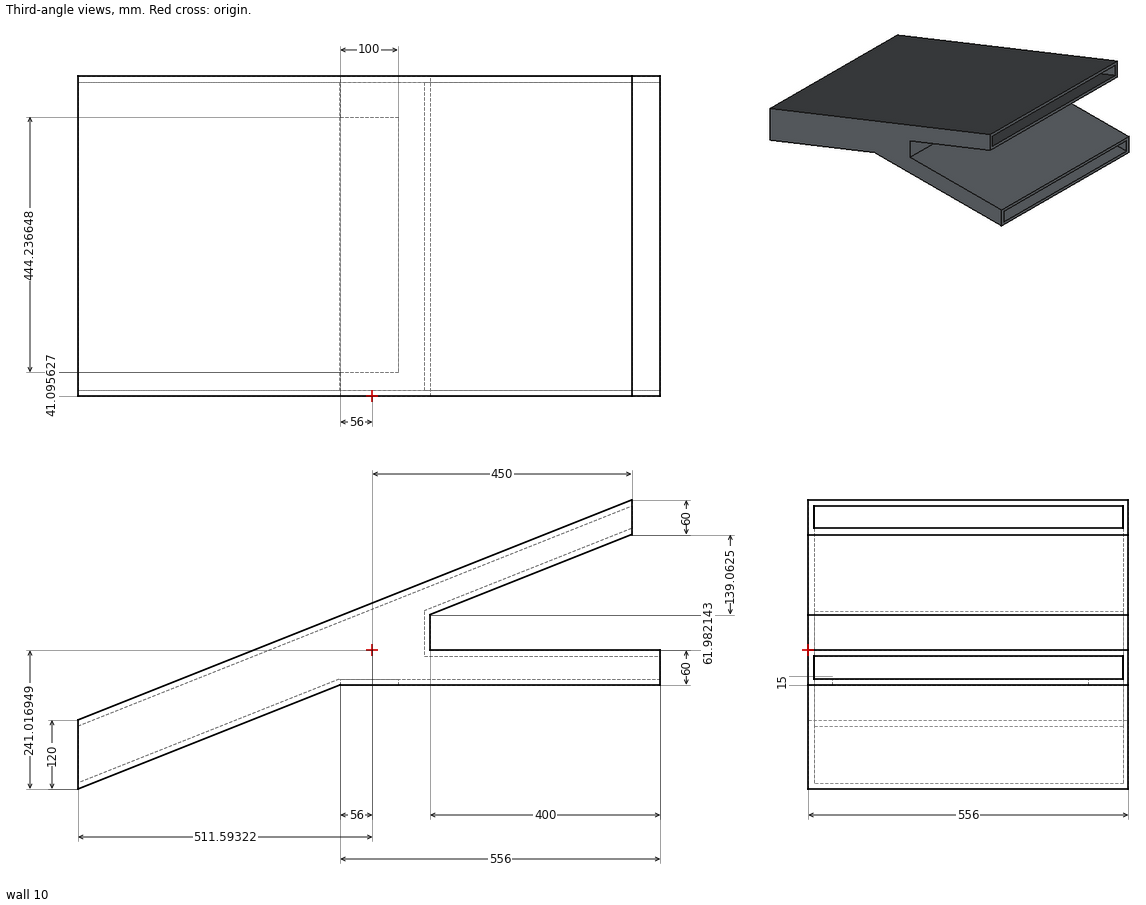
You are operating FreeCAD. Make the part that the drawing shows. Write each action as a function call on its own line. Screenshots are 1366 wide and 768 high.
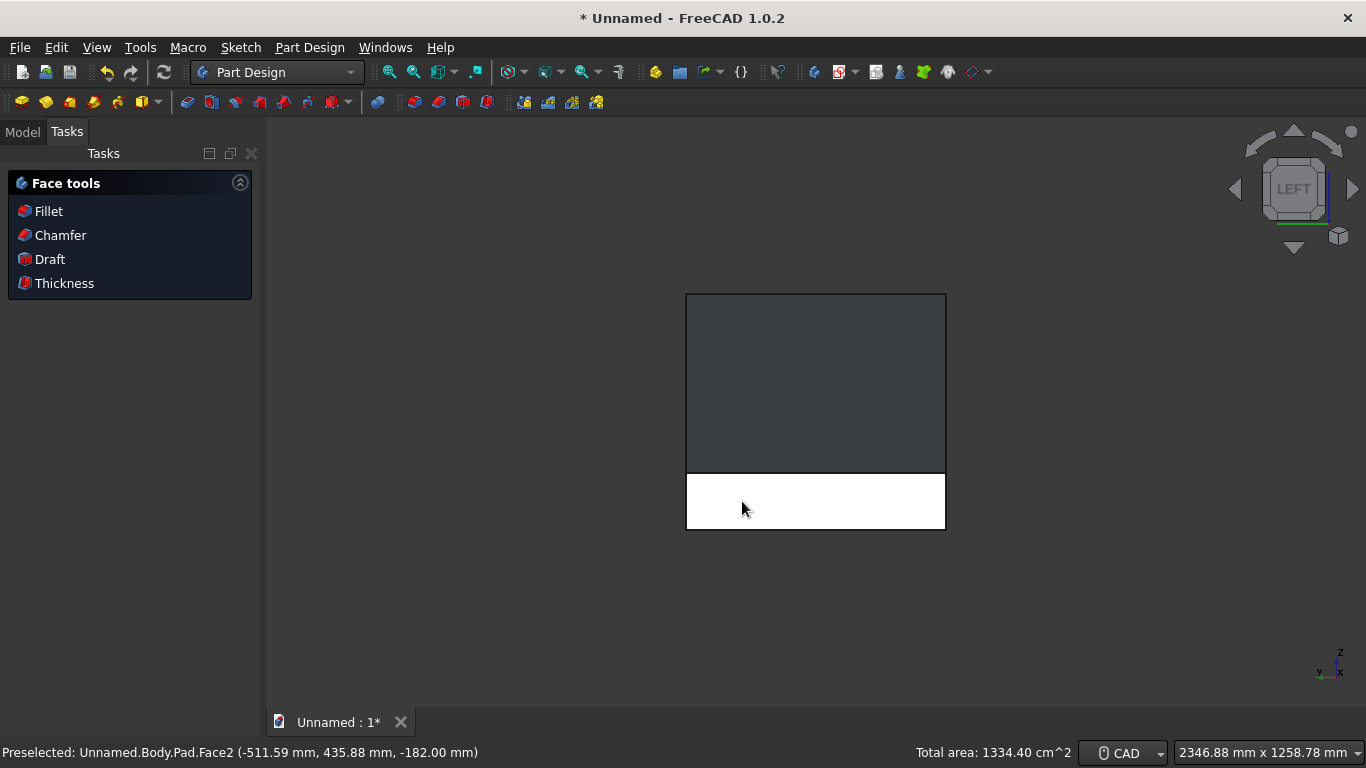
click(488, 102)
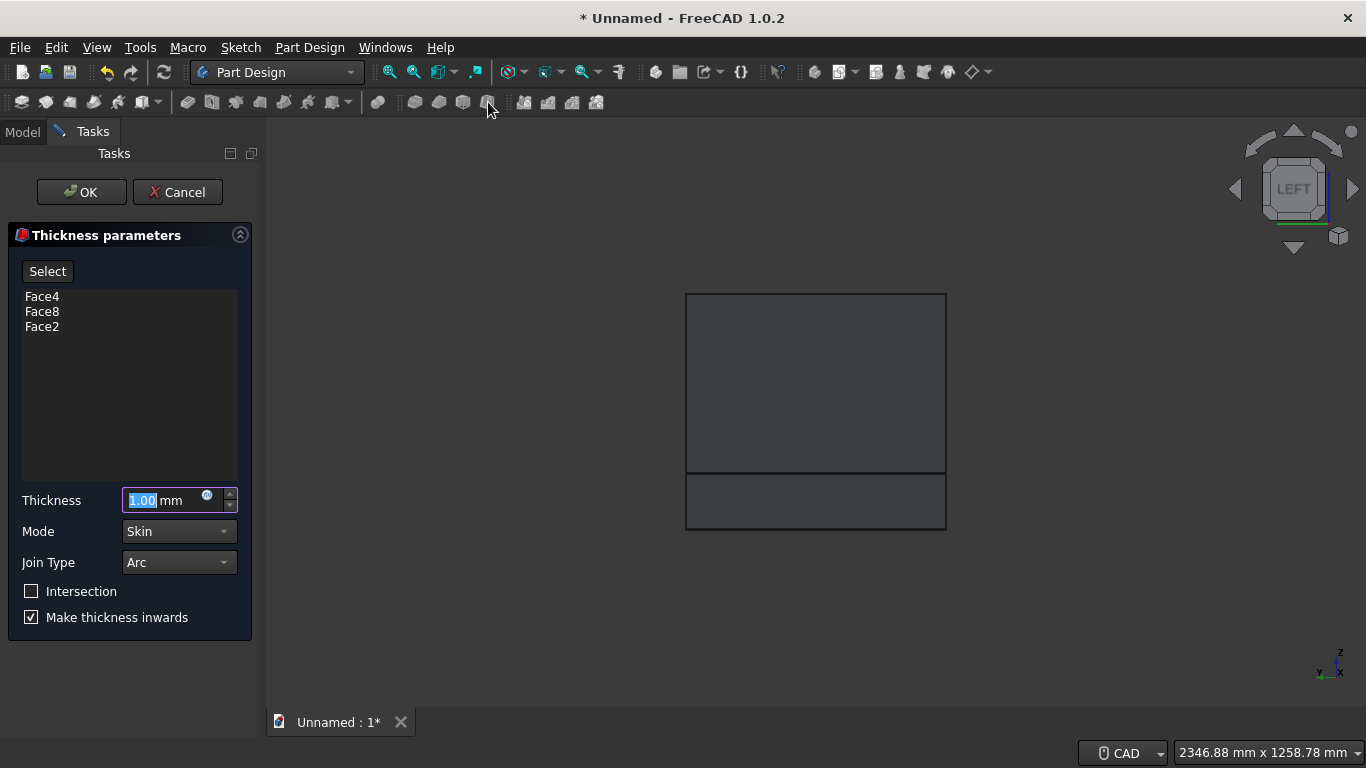
text(10)
key(Tab)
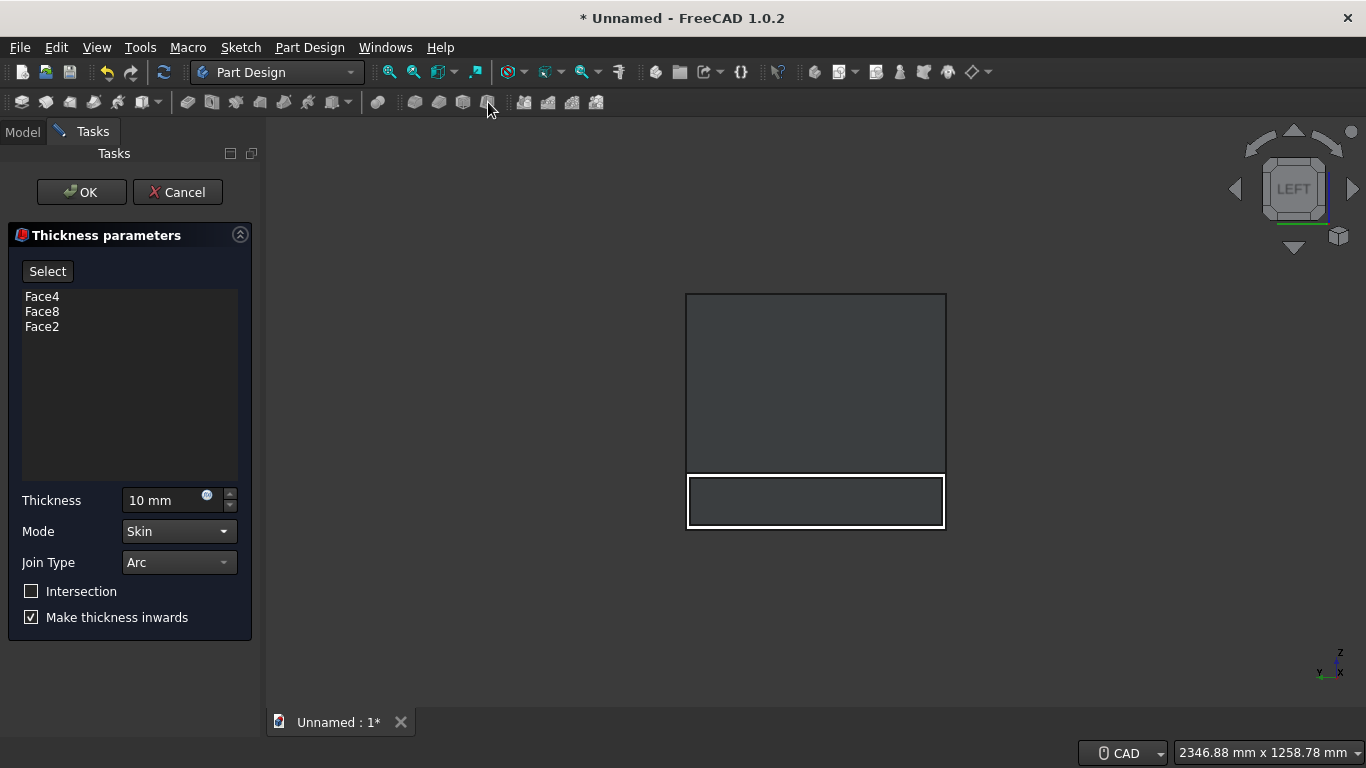
click(180, 562)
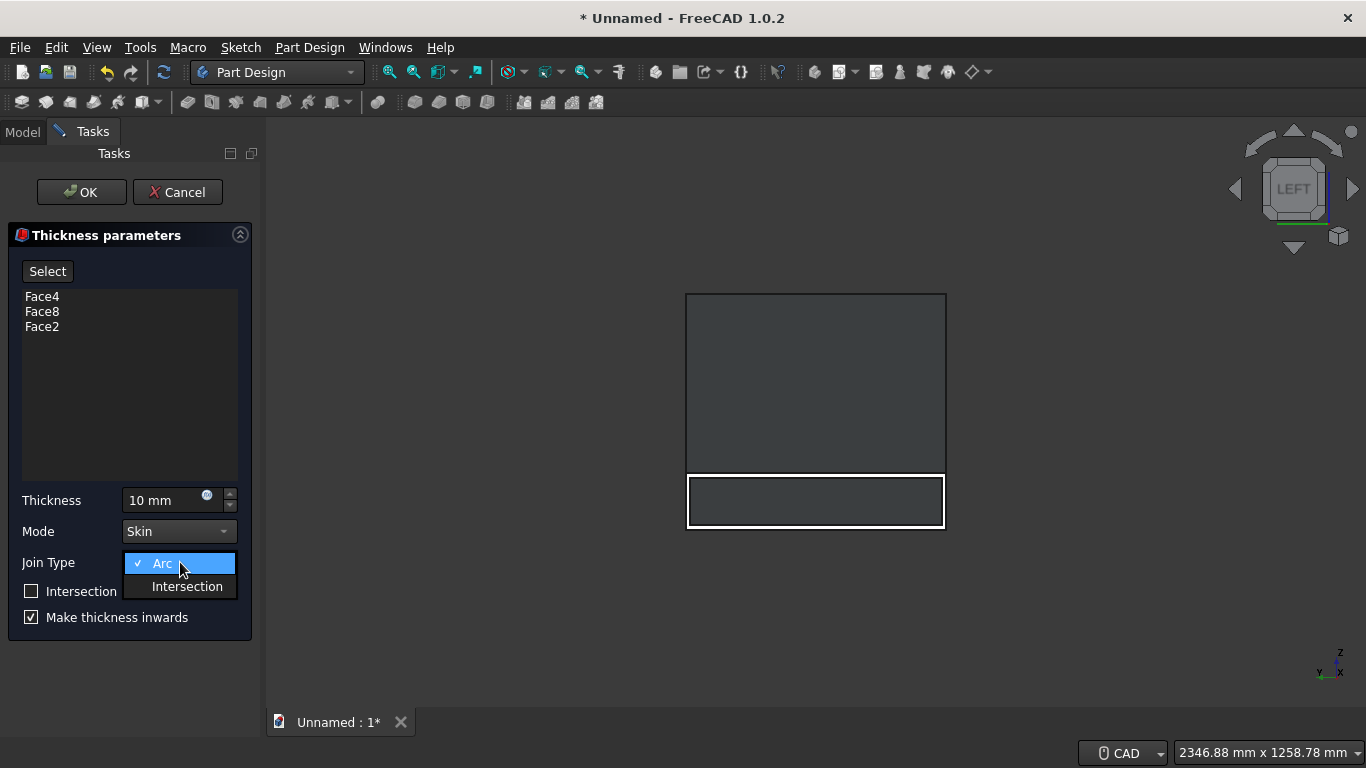
click(179, 586)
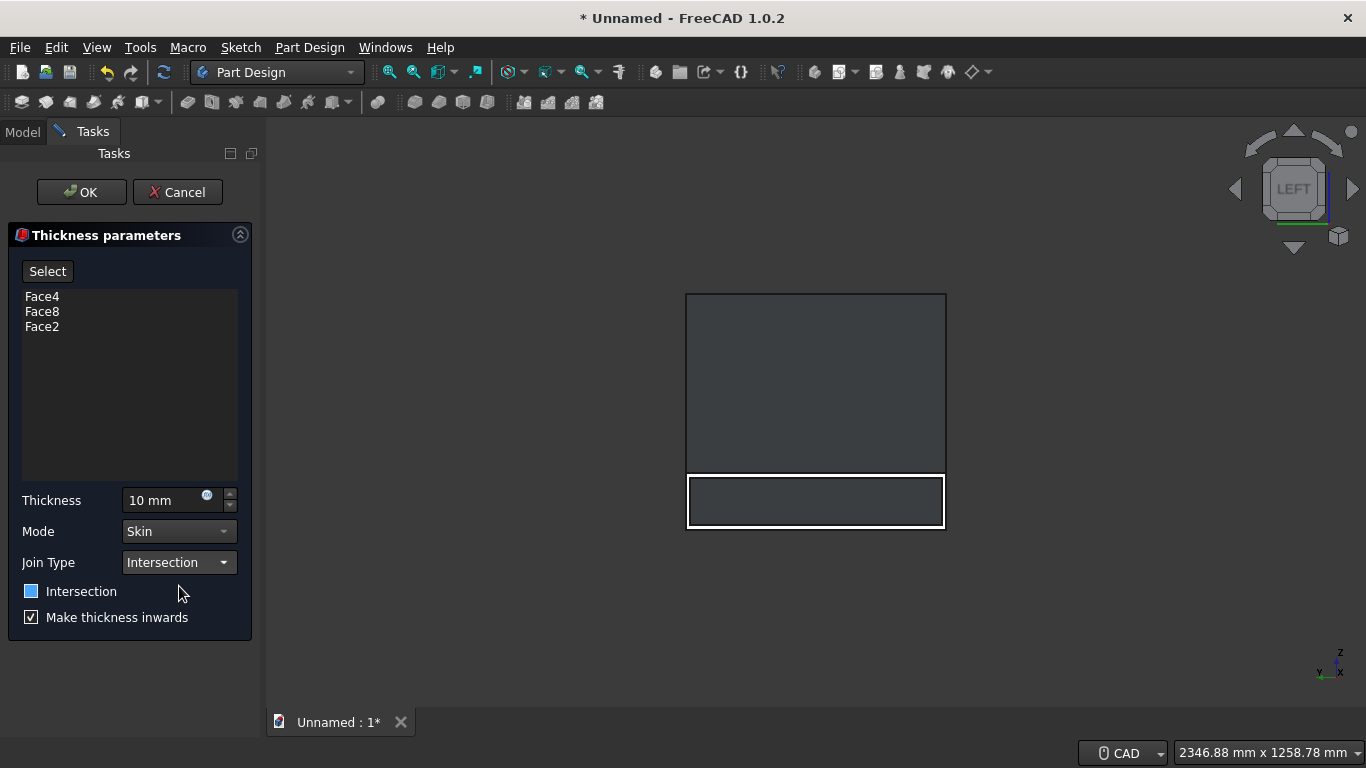
click(82, 192)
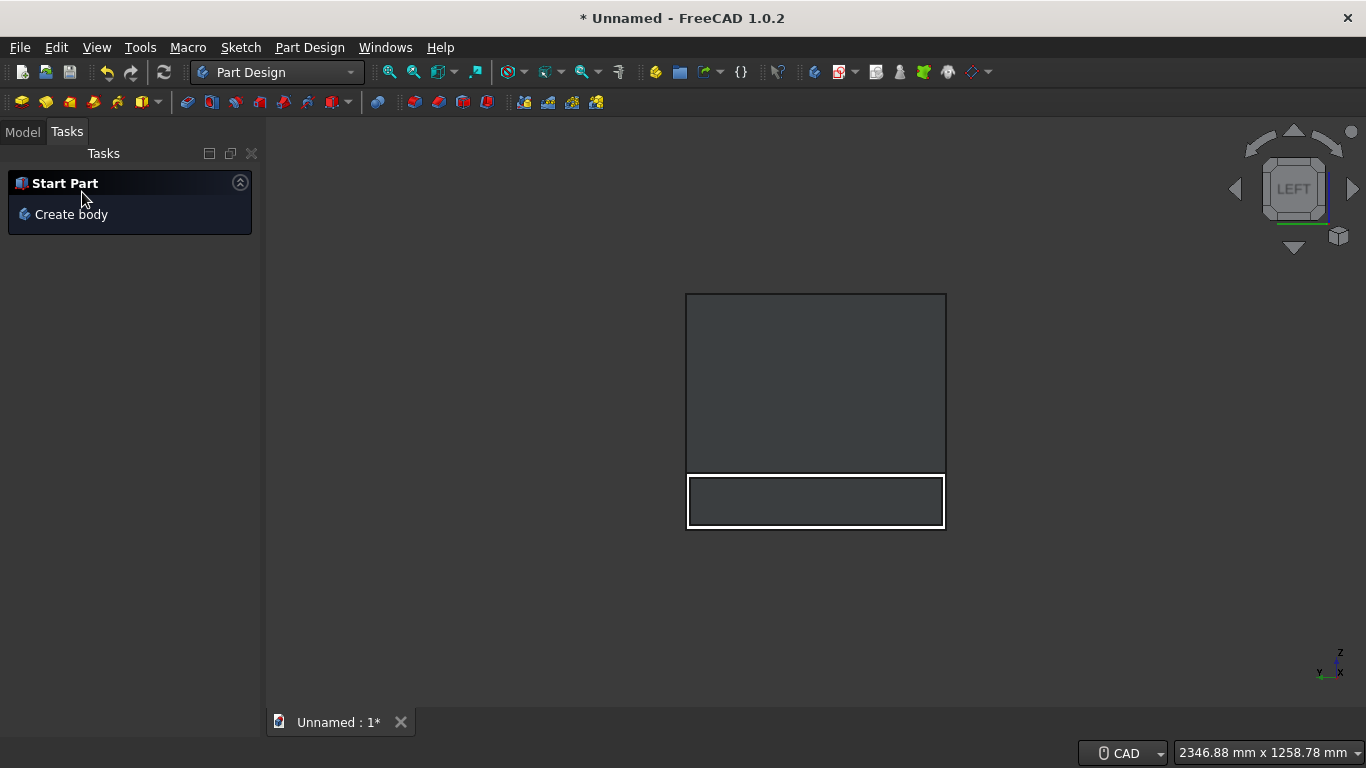
click(390, 72)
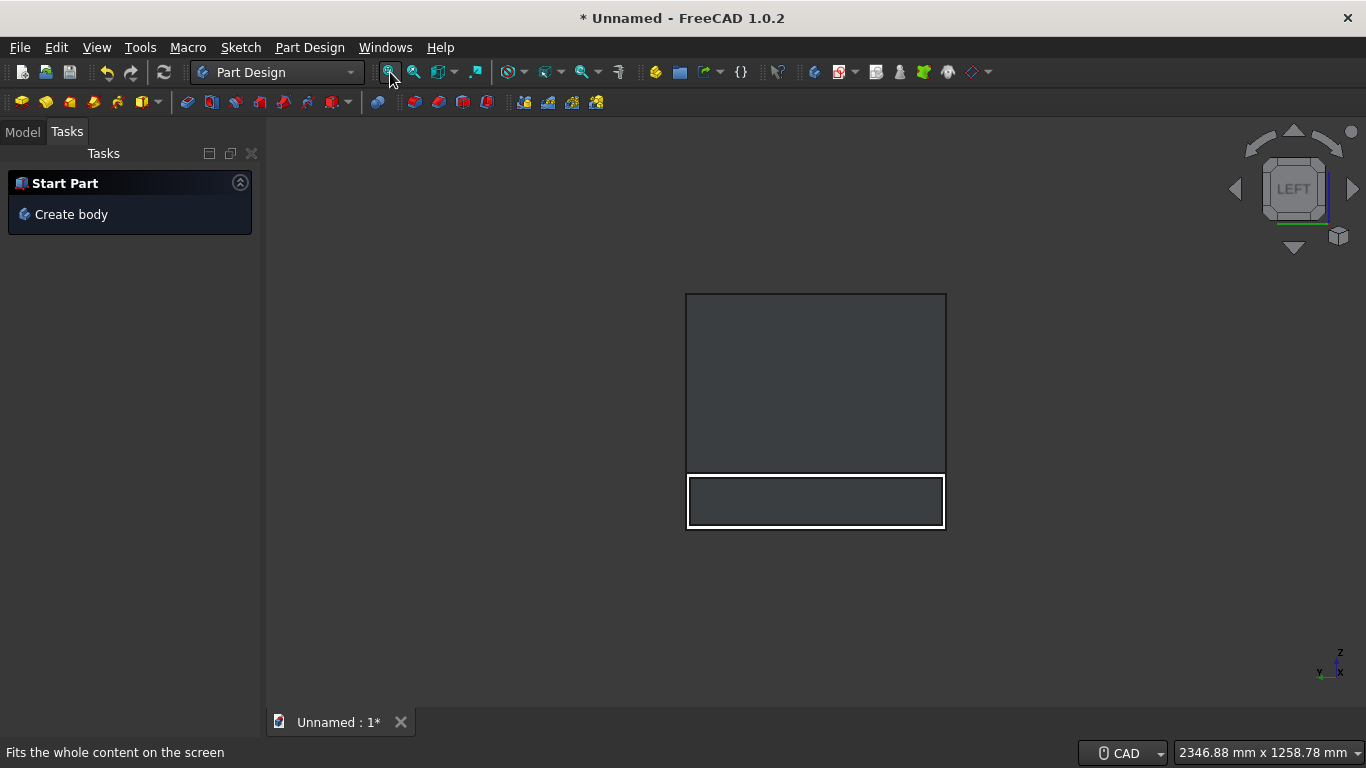
key(5)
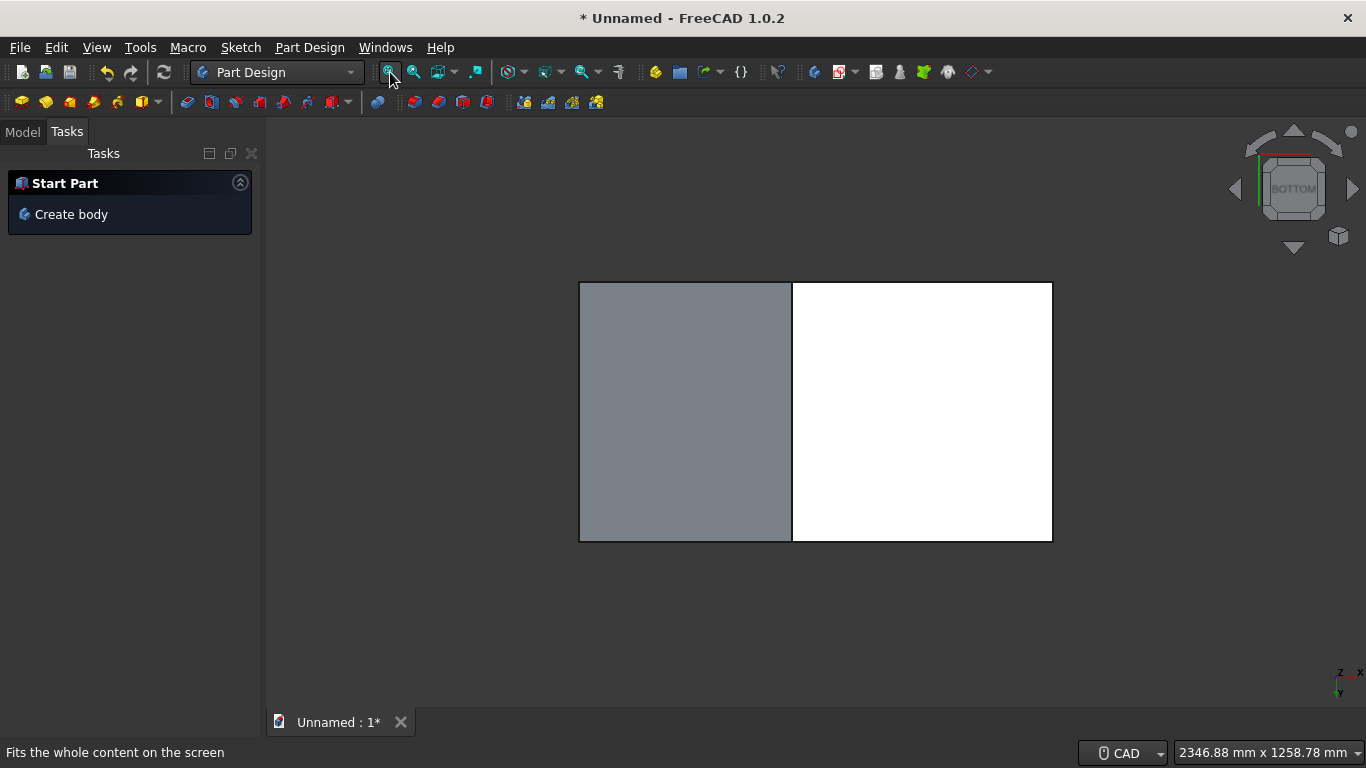
click(390, 72)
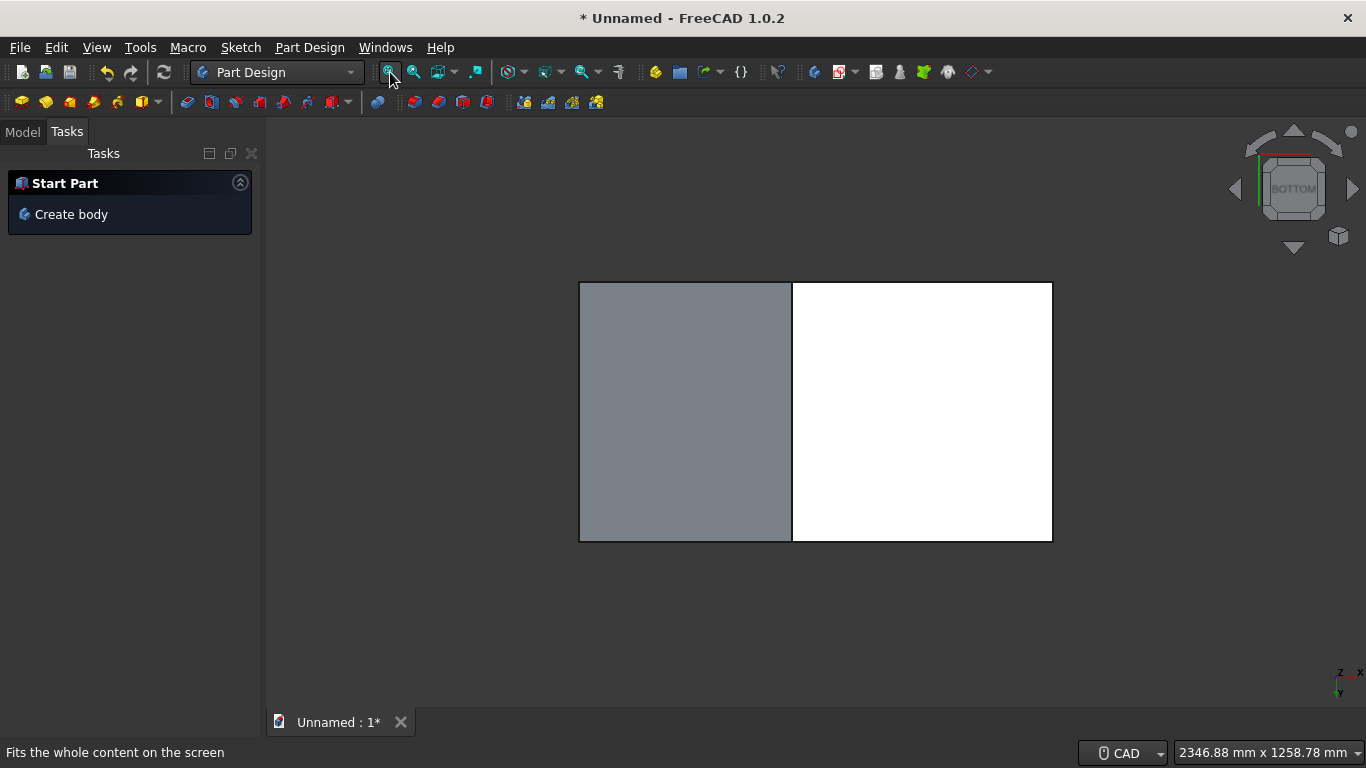
click(923, 411)